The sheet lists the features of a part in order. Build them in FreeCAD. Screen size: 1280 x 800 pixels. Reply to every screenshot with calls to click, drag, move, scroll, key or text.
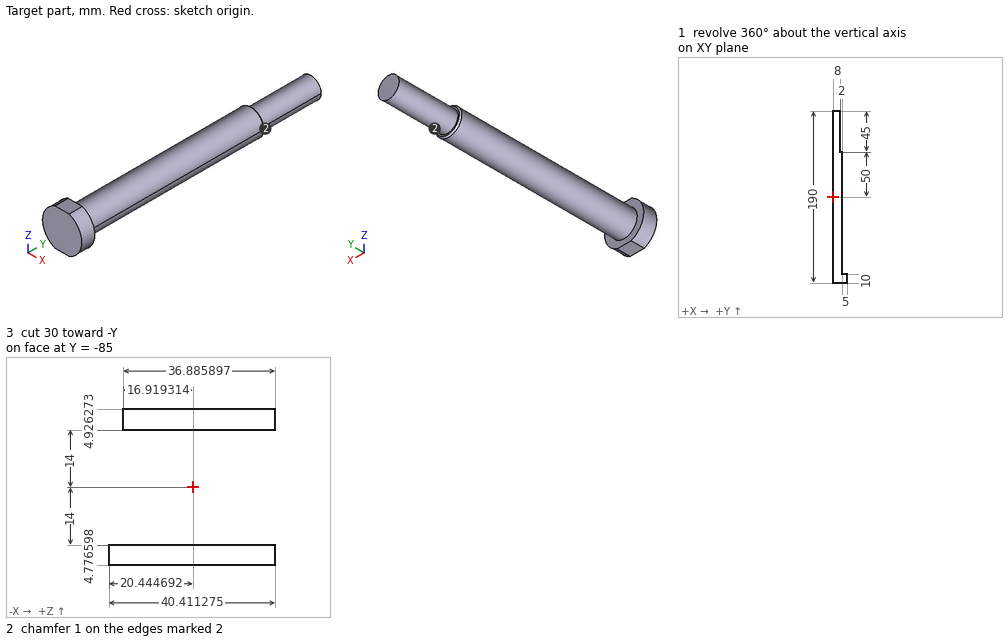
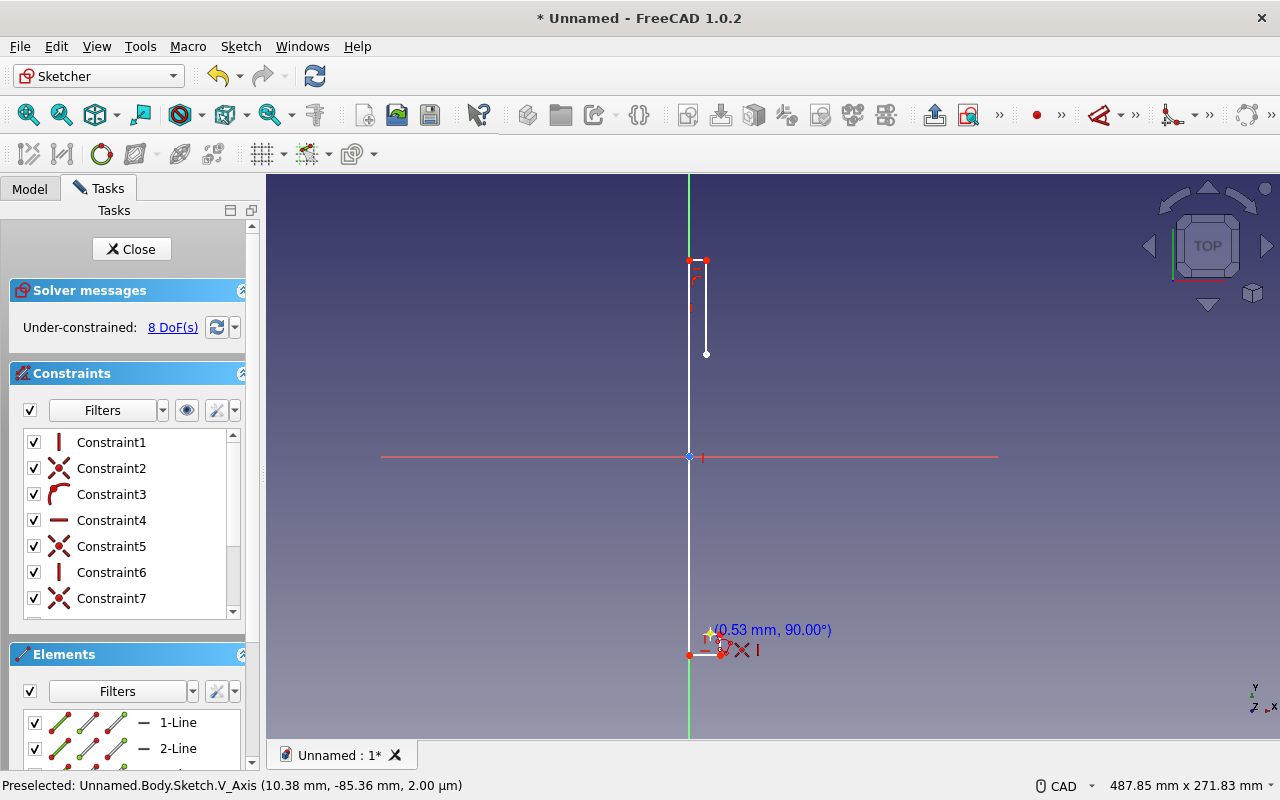
scroll(710, 353, up, 7)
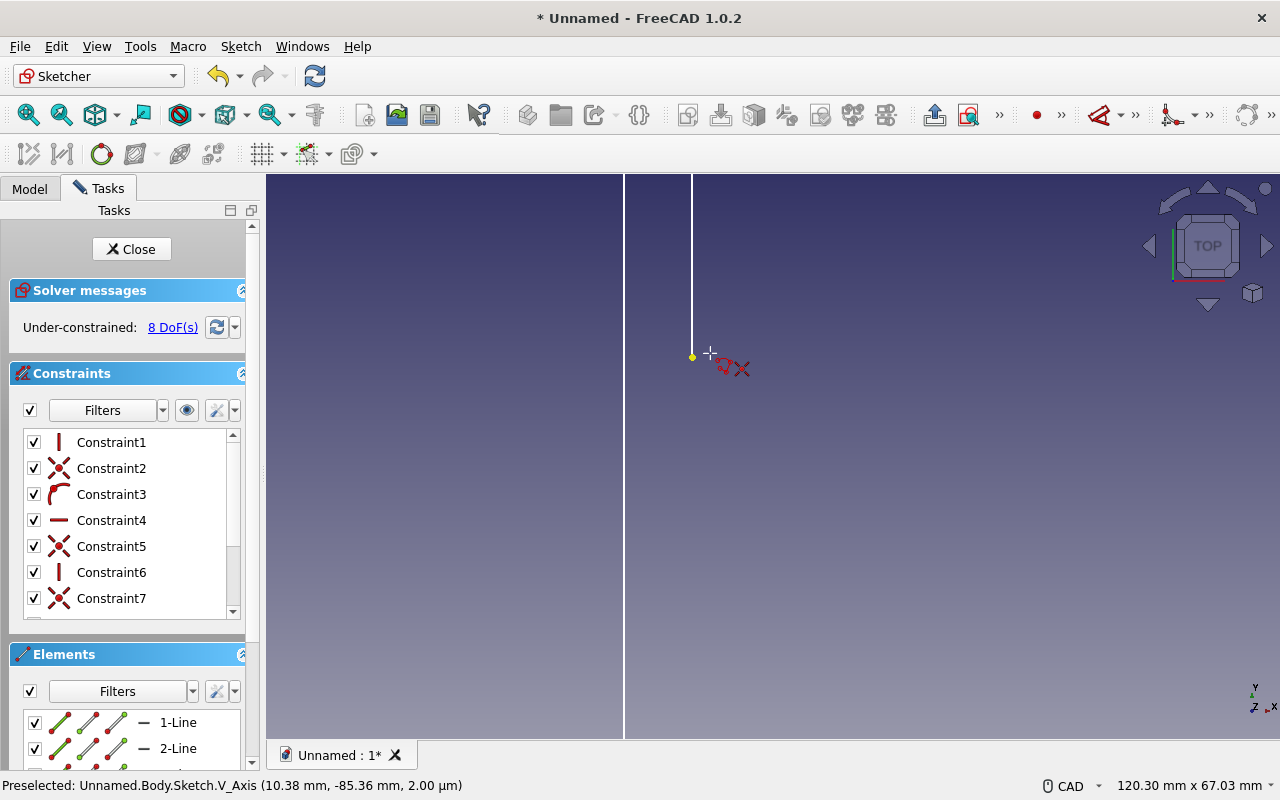
click(709, 352)
click(692, 358)
key(Escape)
key(Escape)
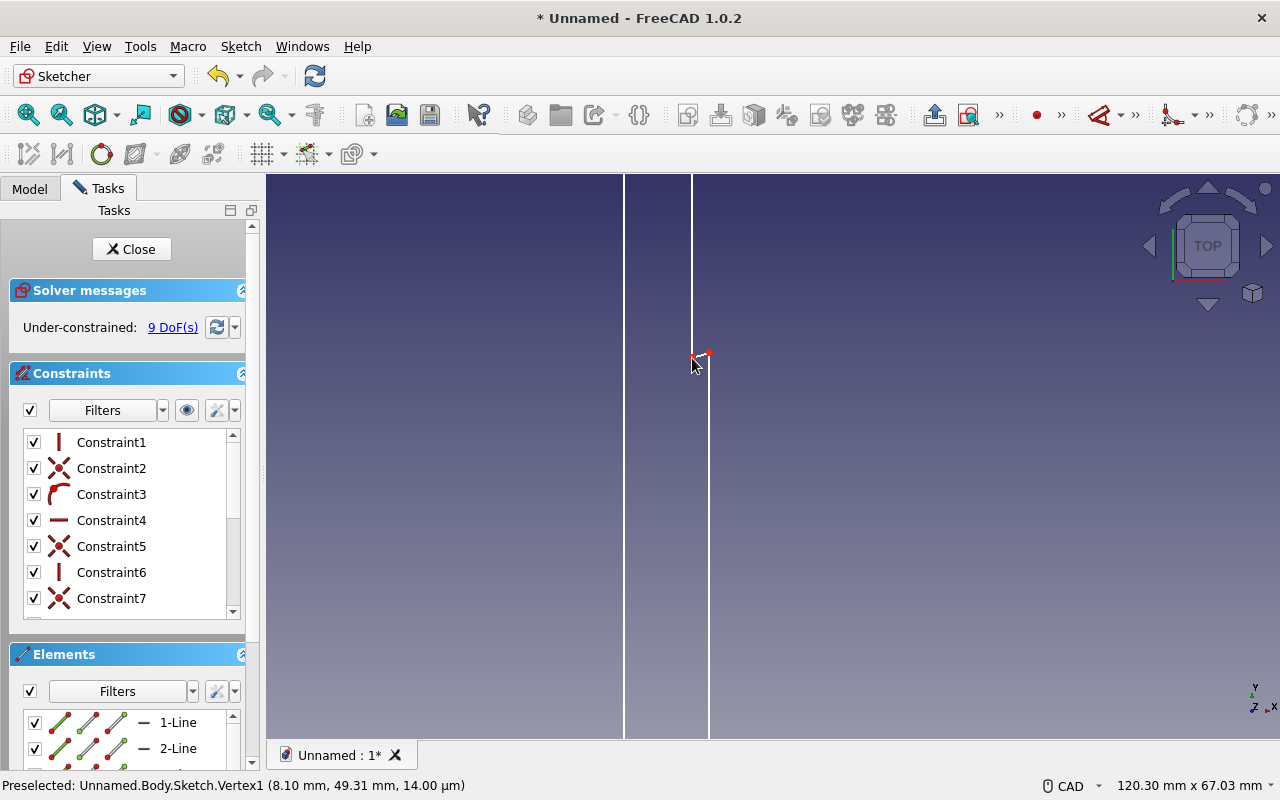
scroll(710, 353, down, 7)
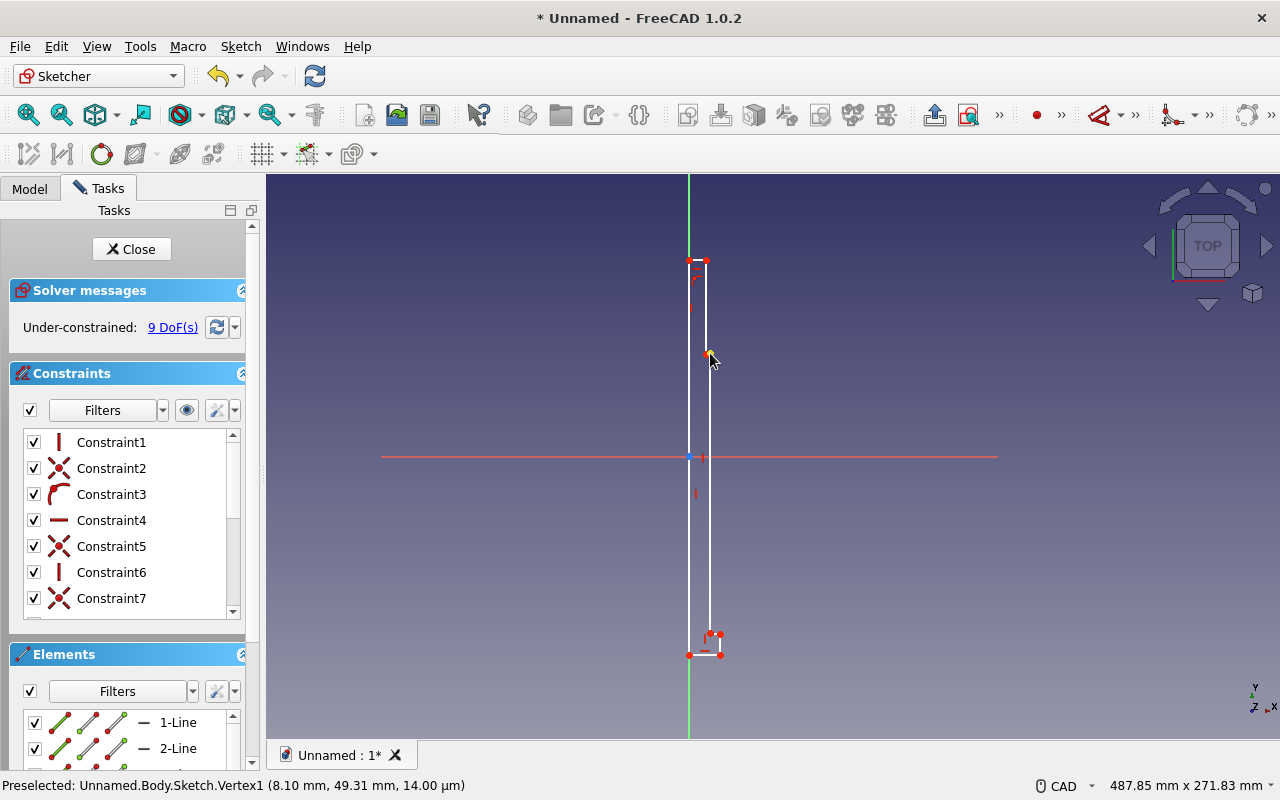
scroll(717, 634, up, 8)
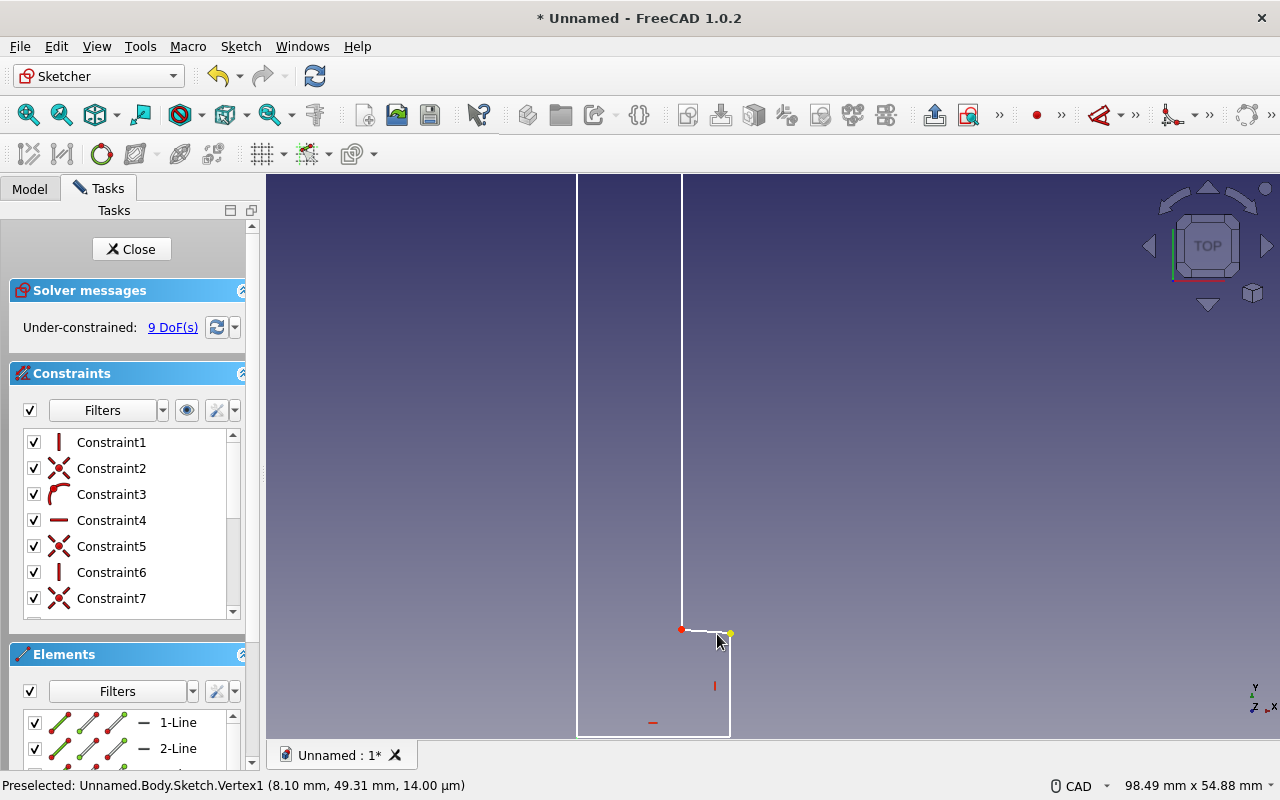
click(716, 632)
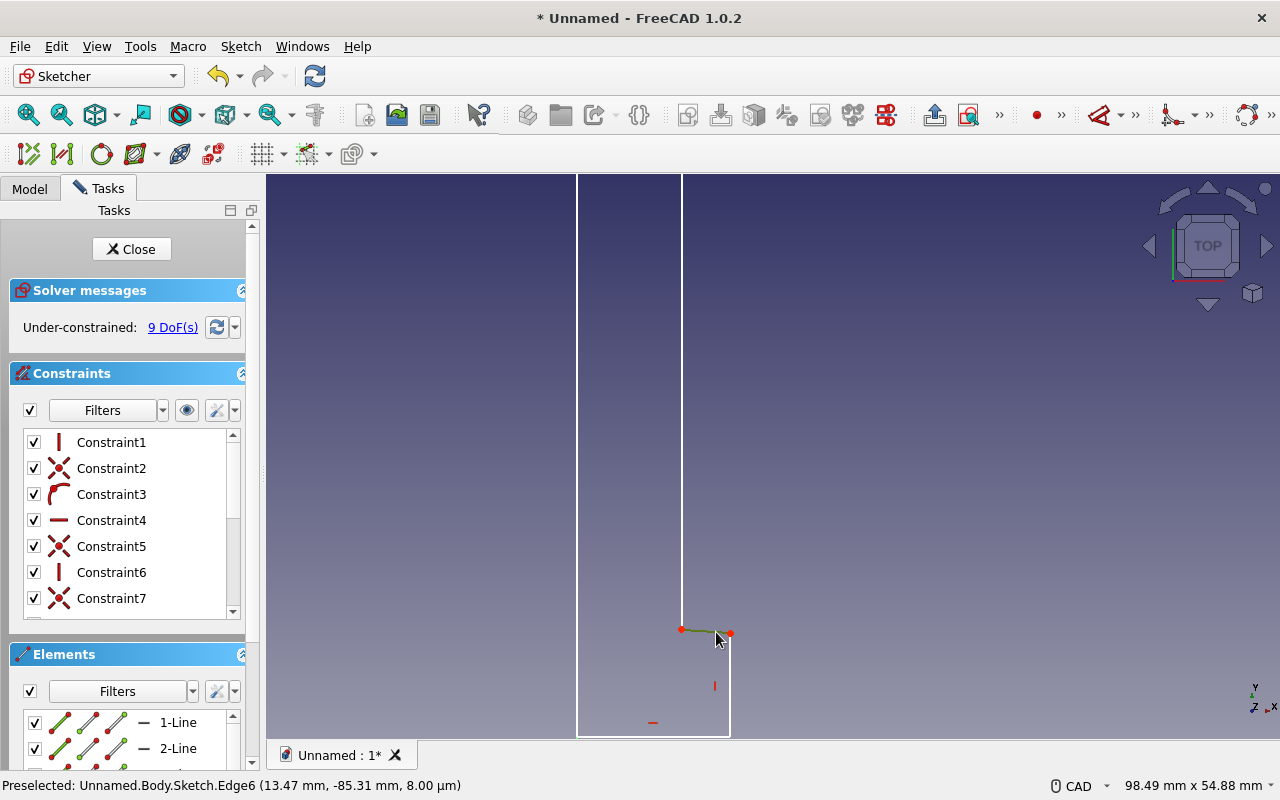
key(h)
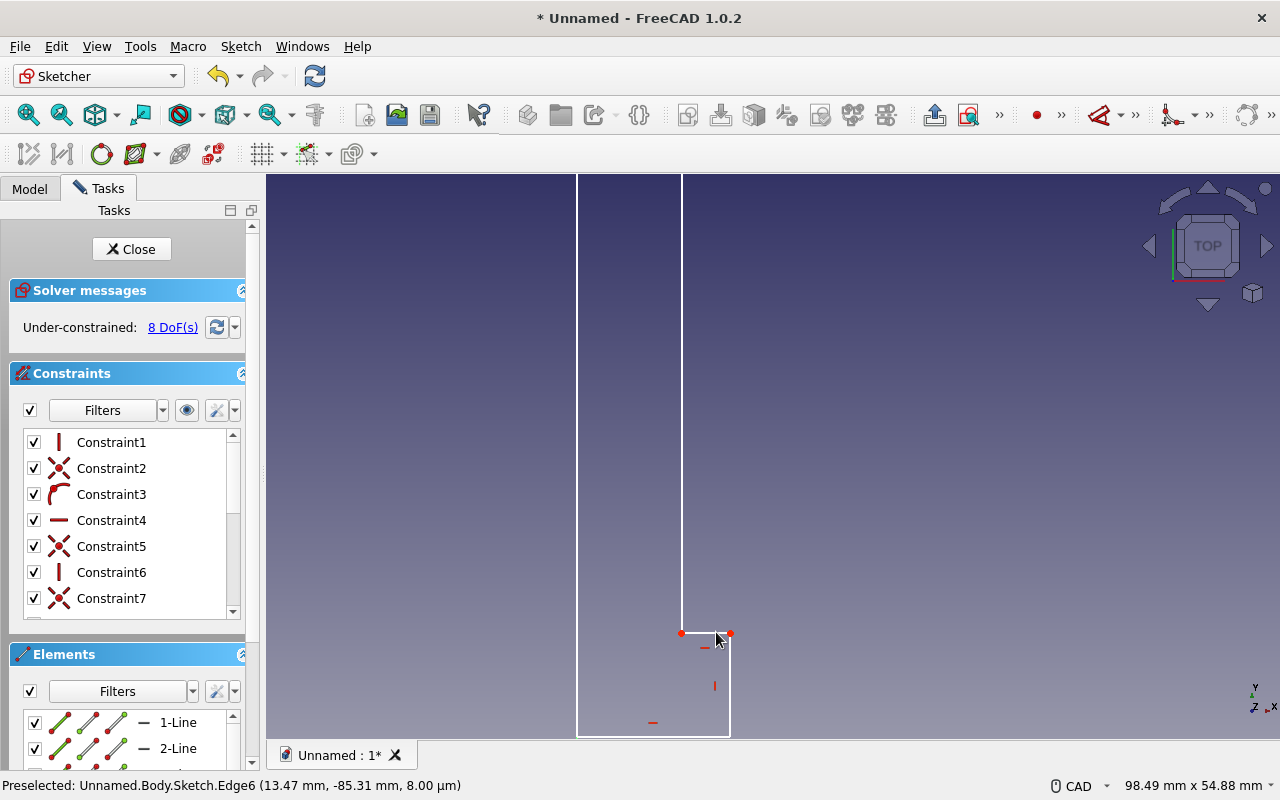
scroll(717, 634, down, 8)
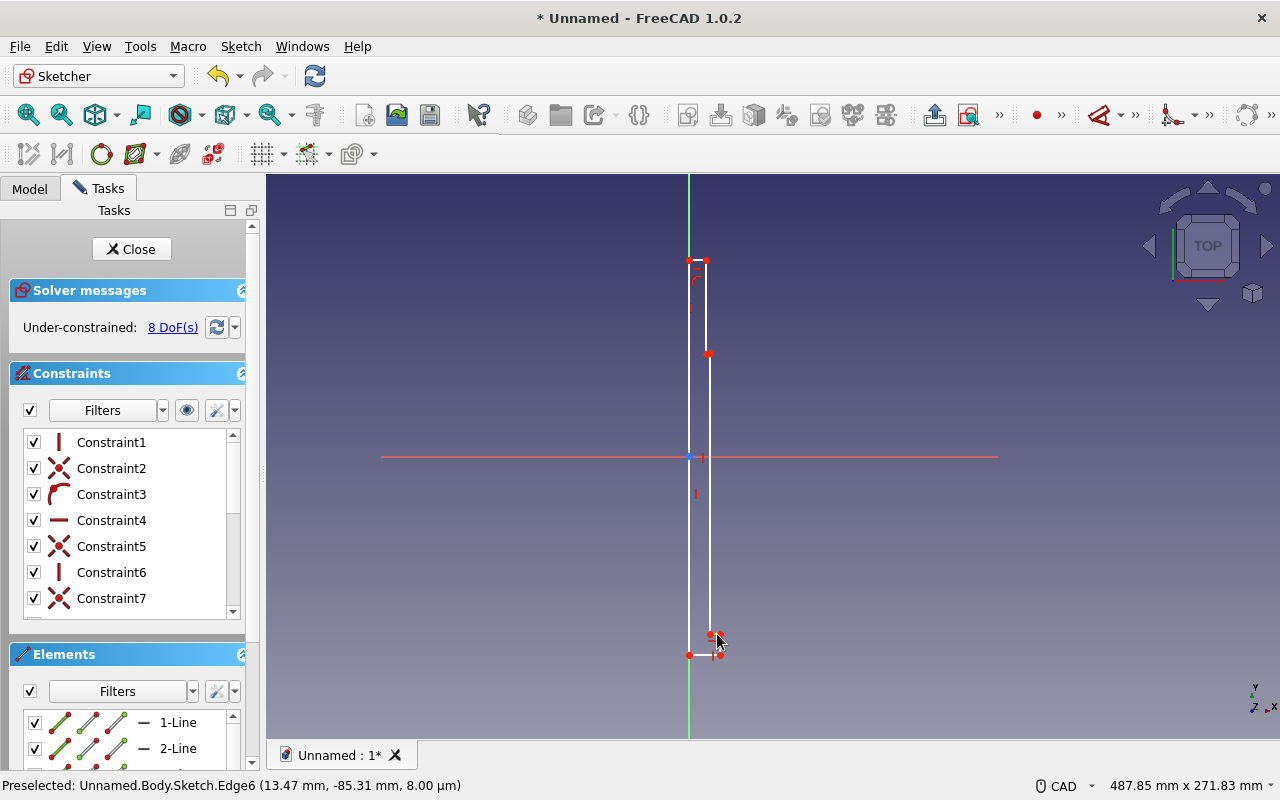
scroll(708, 354, up, 10)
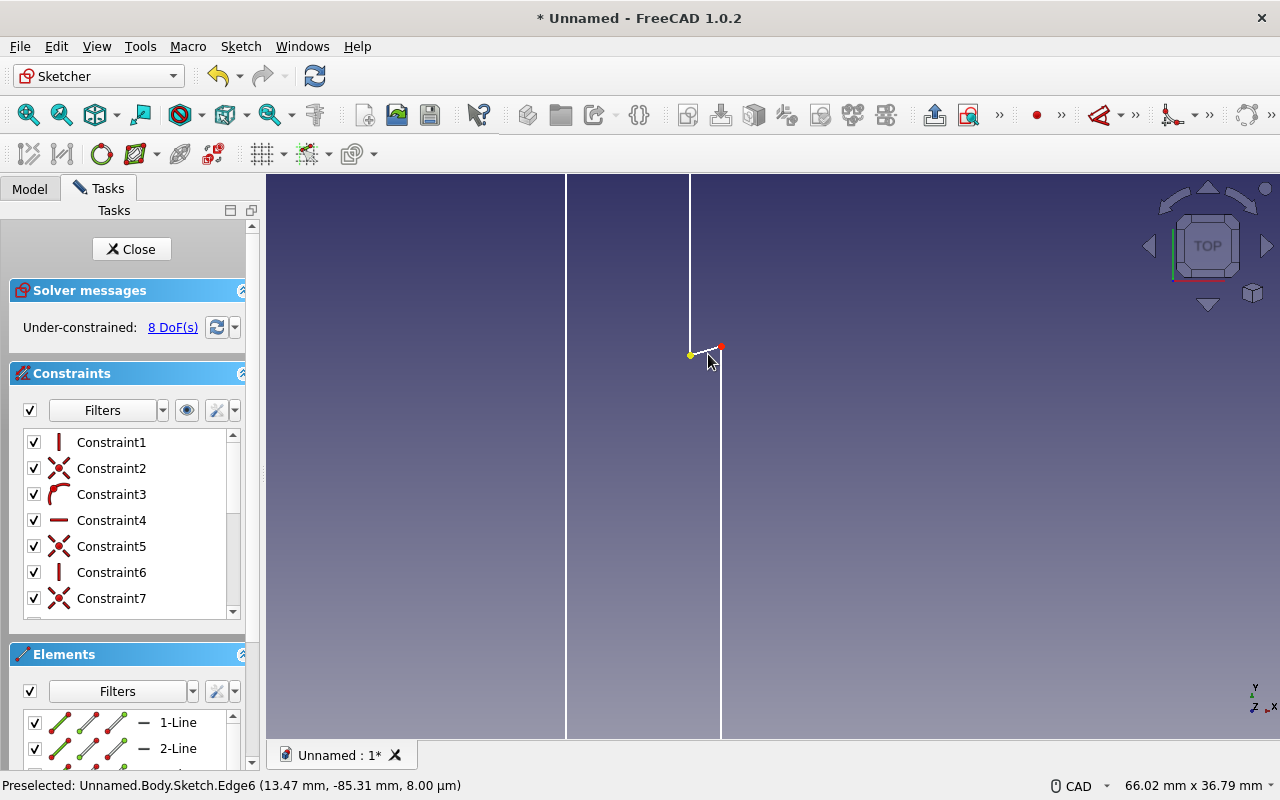
click(706, 351)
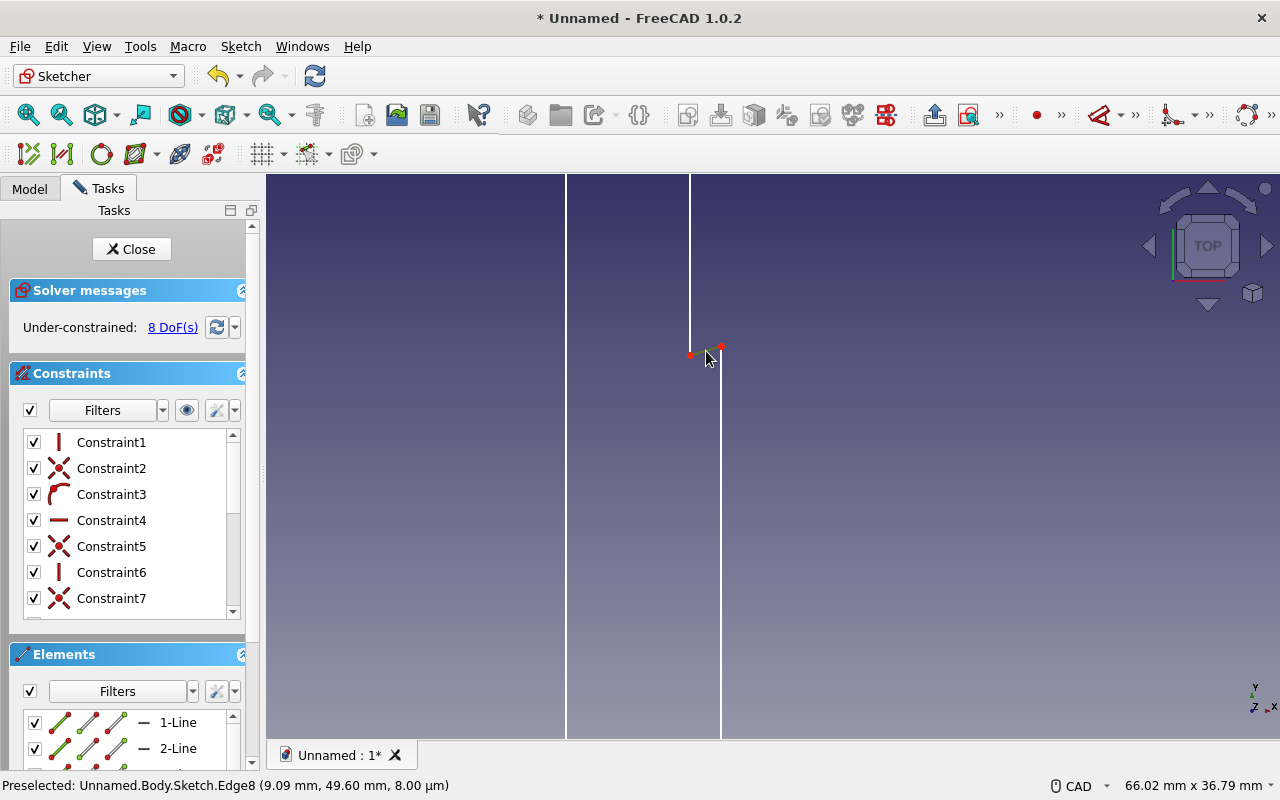
key(h)